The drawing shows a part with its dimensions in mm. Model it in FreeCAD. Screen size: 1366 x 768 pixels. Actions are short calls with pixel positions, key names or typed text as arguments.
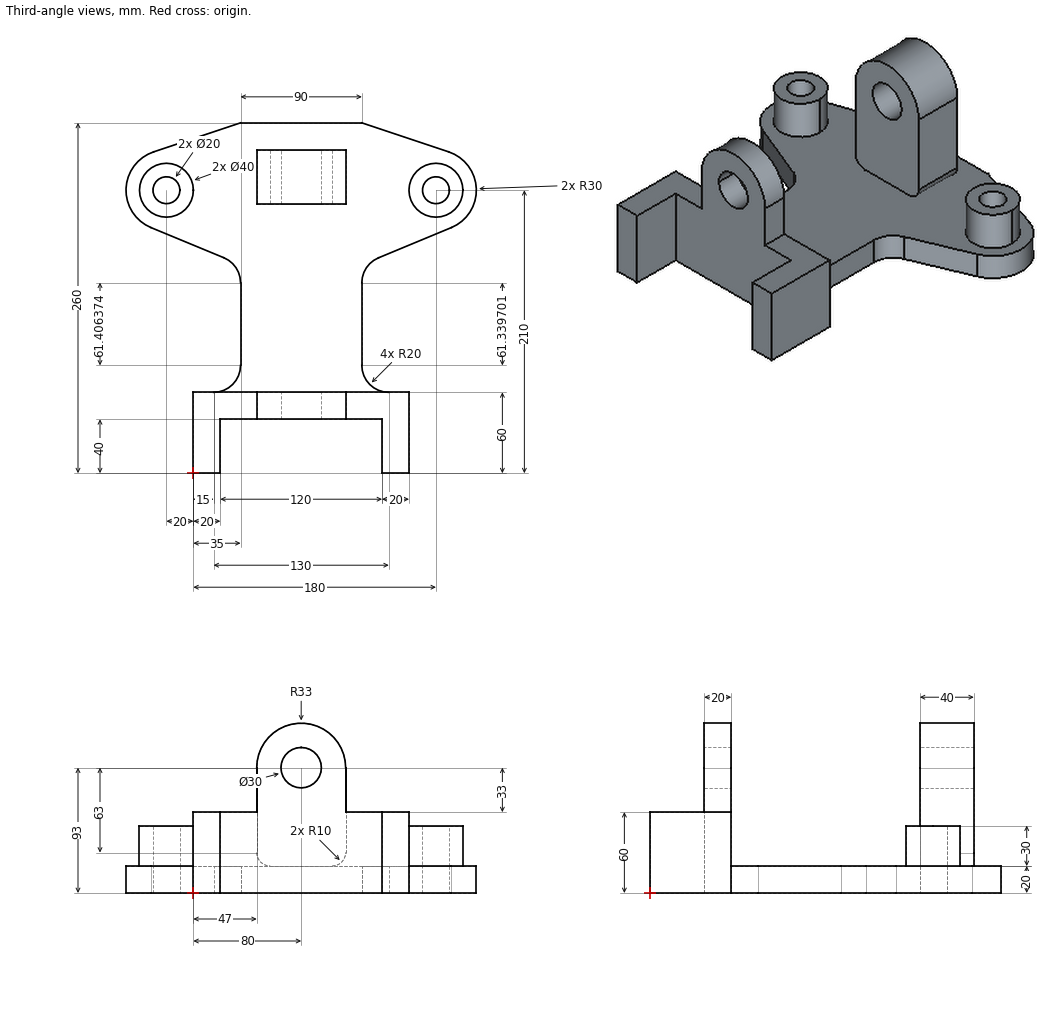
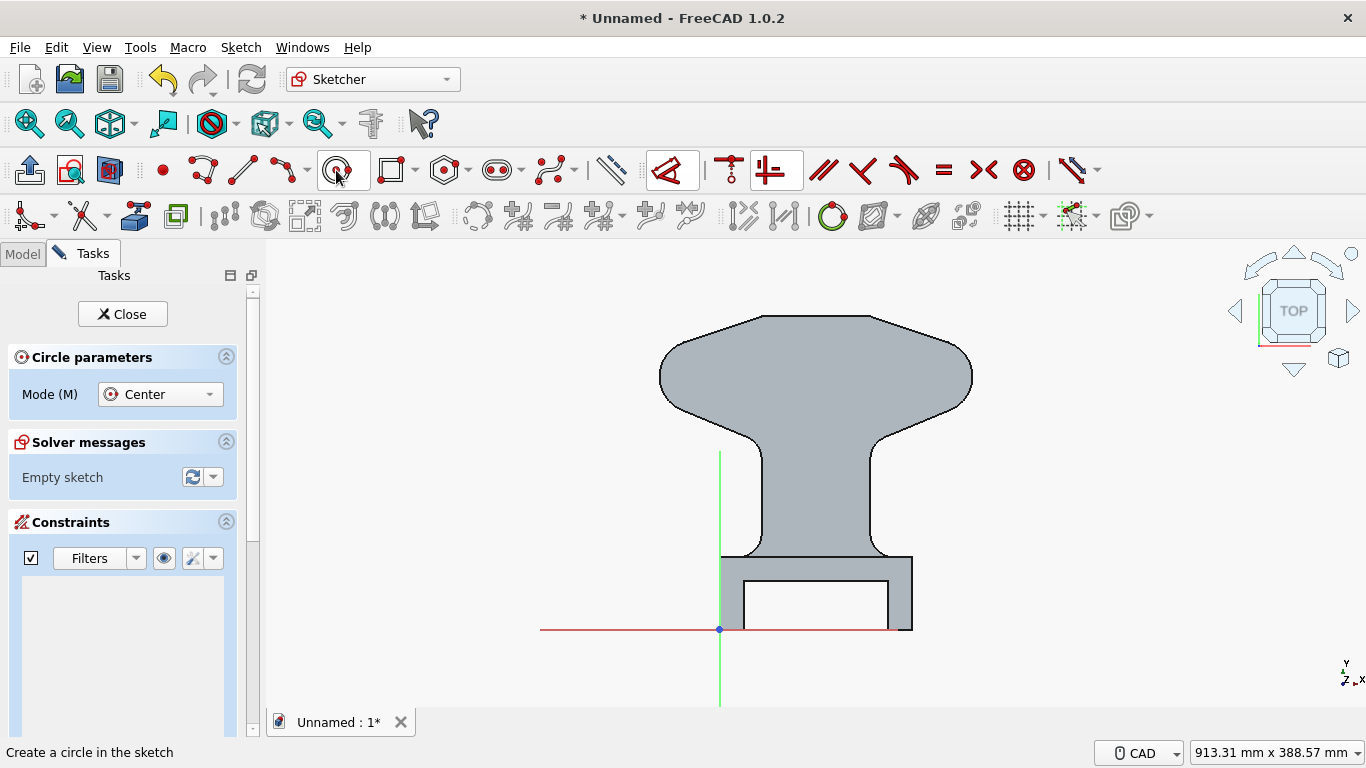
click(696, 377)
click(679, 360)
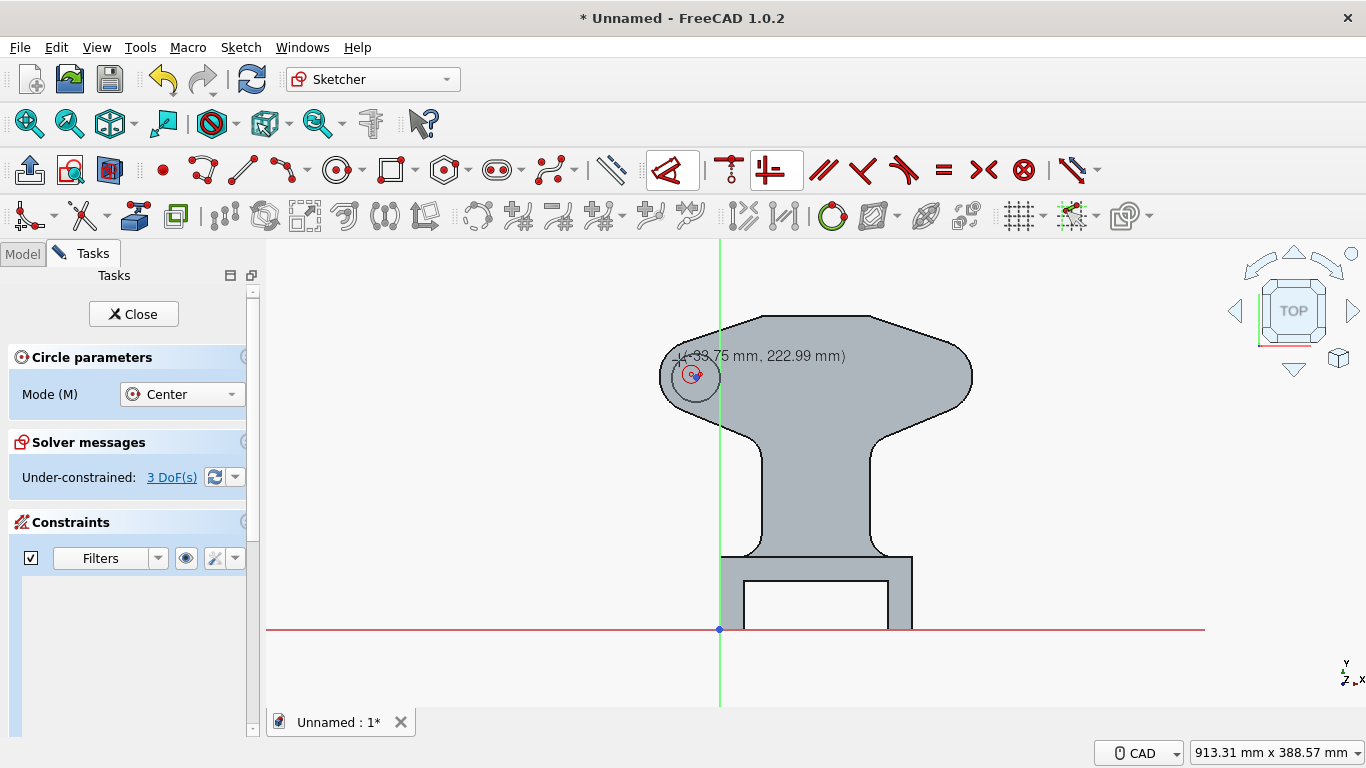
click(936, 377)
click(953, 360)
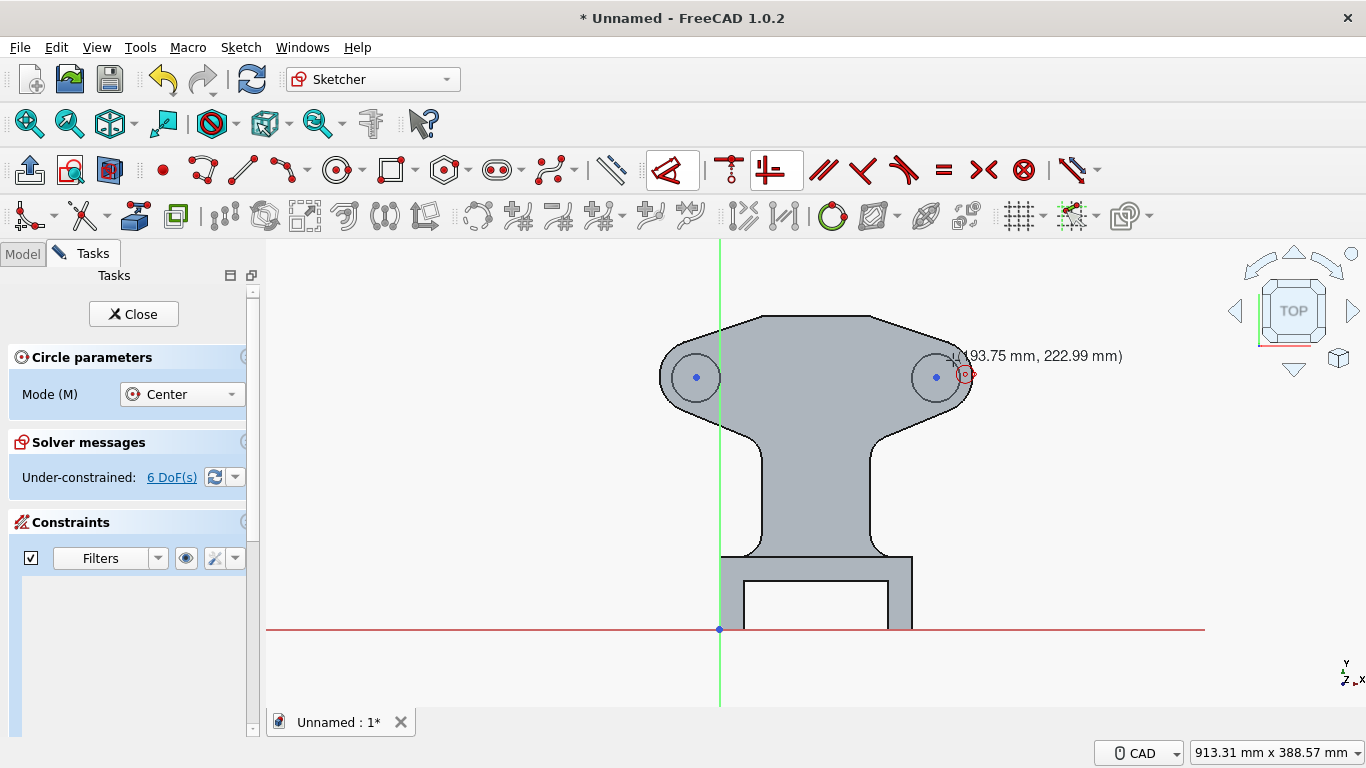
scroll(696, 377, up, 4)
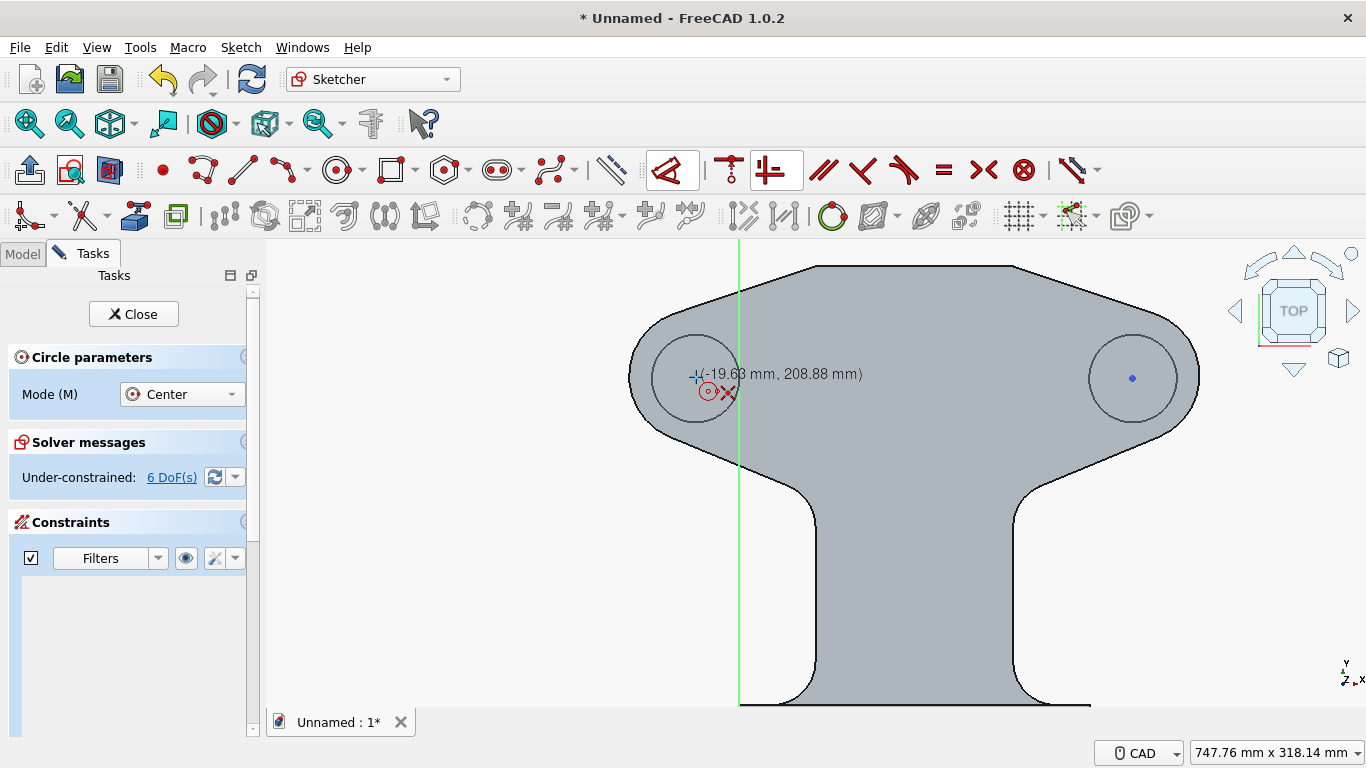
click(696, 379)
click(713, 357)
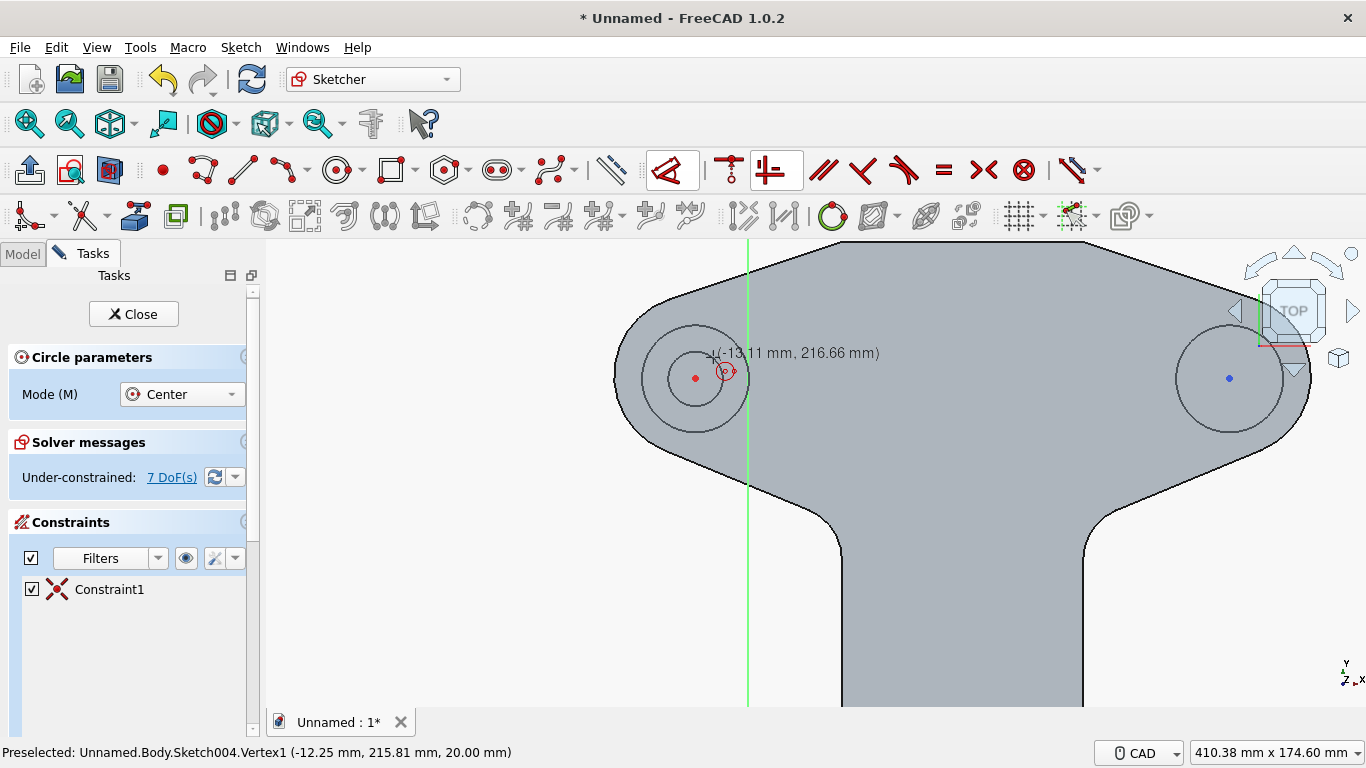
scroll(572, 344, down, 4)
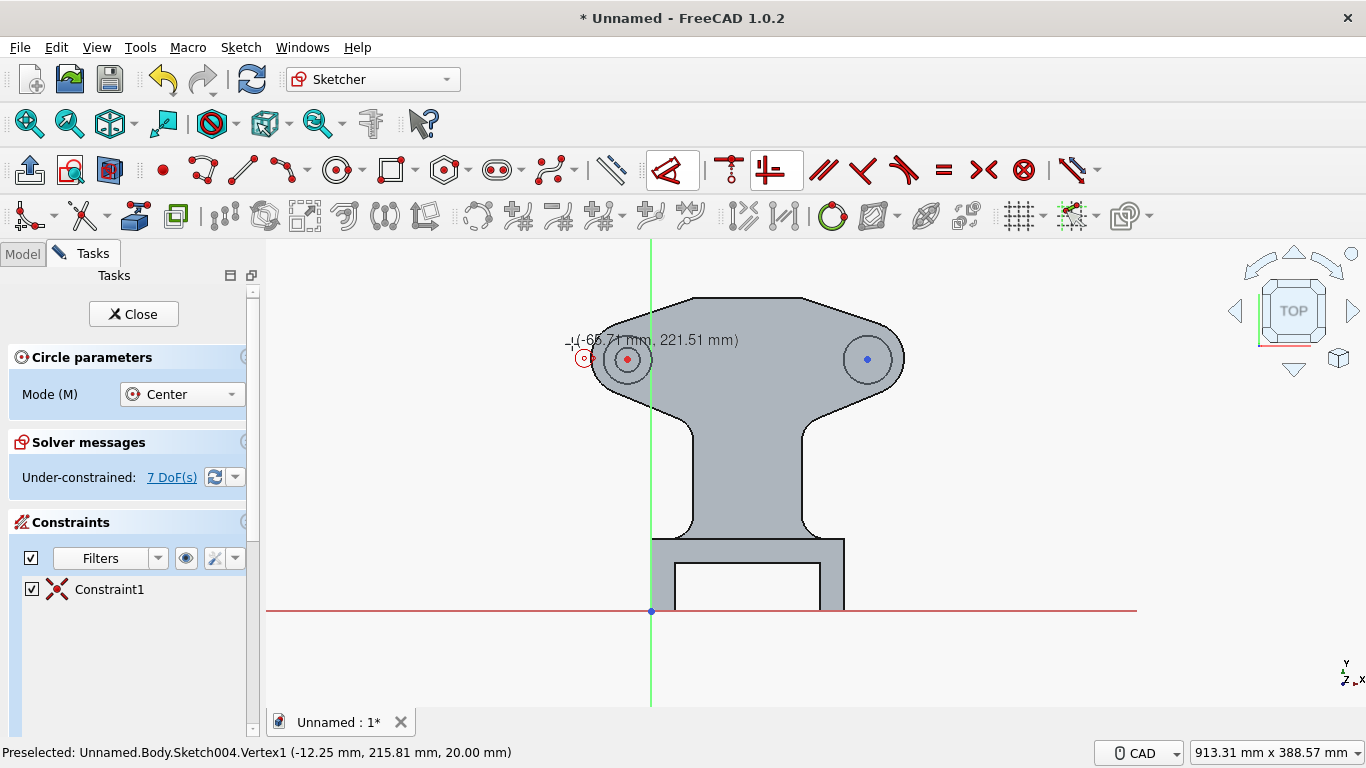
scroll(868, 358, up, 4)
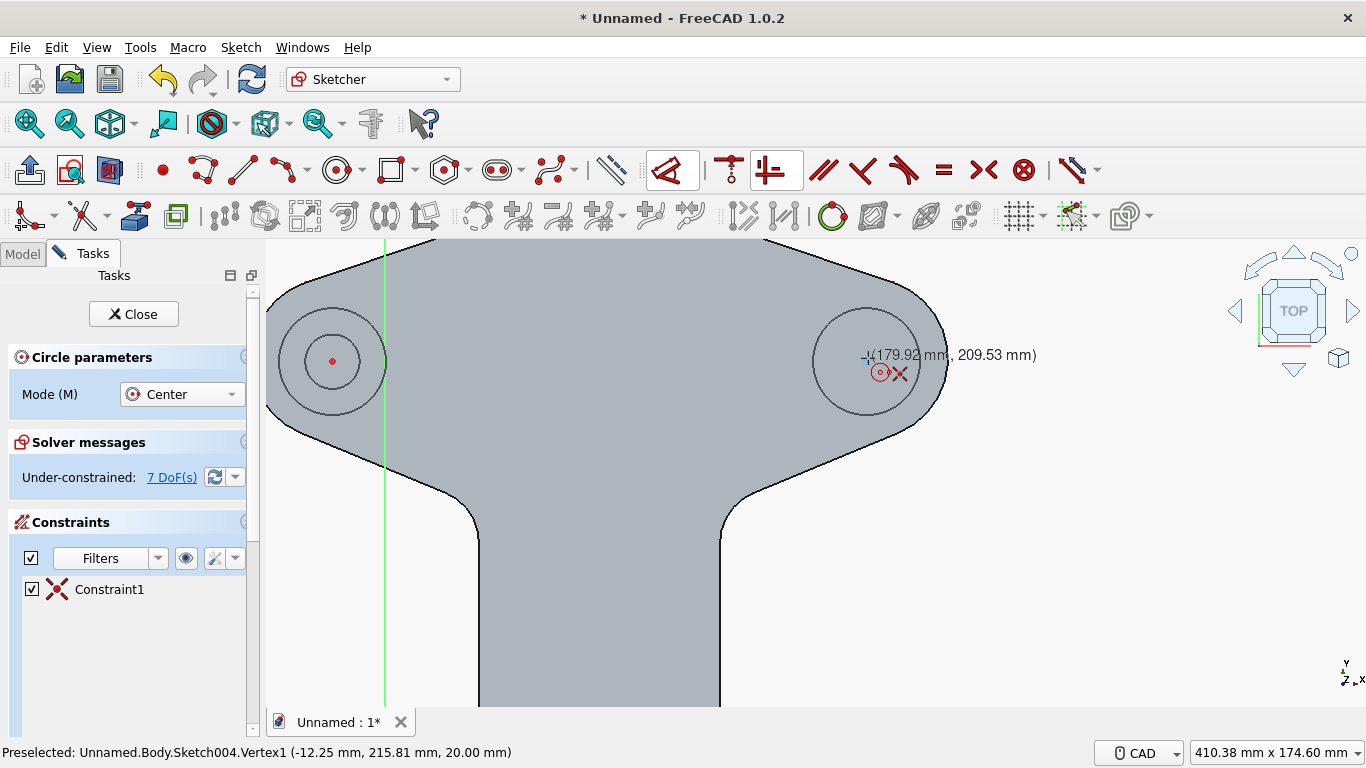
click(867, 362)
click(886, 340)
key(Escape)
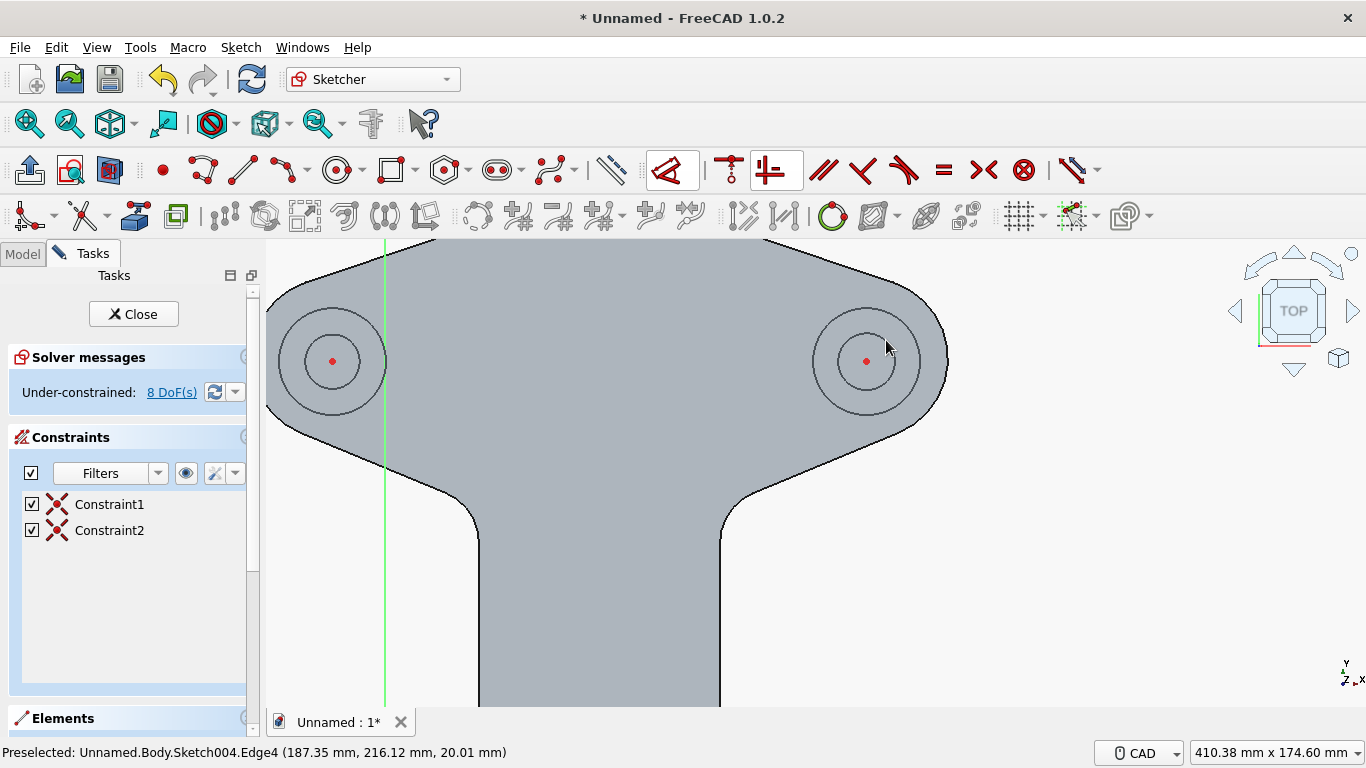
click(370, 324)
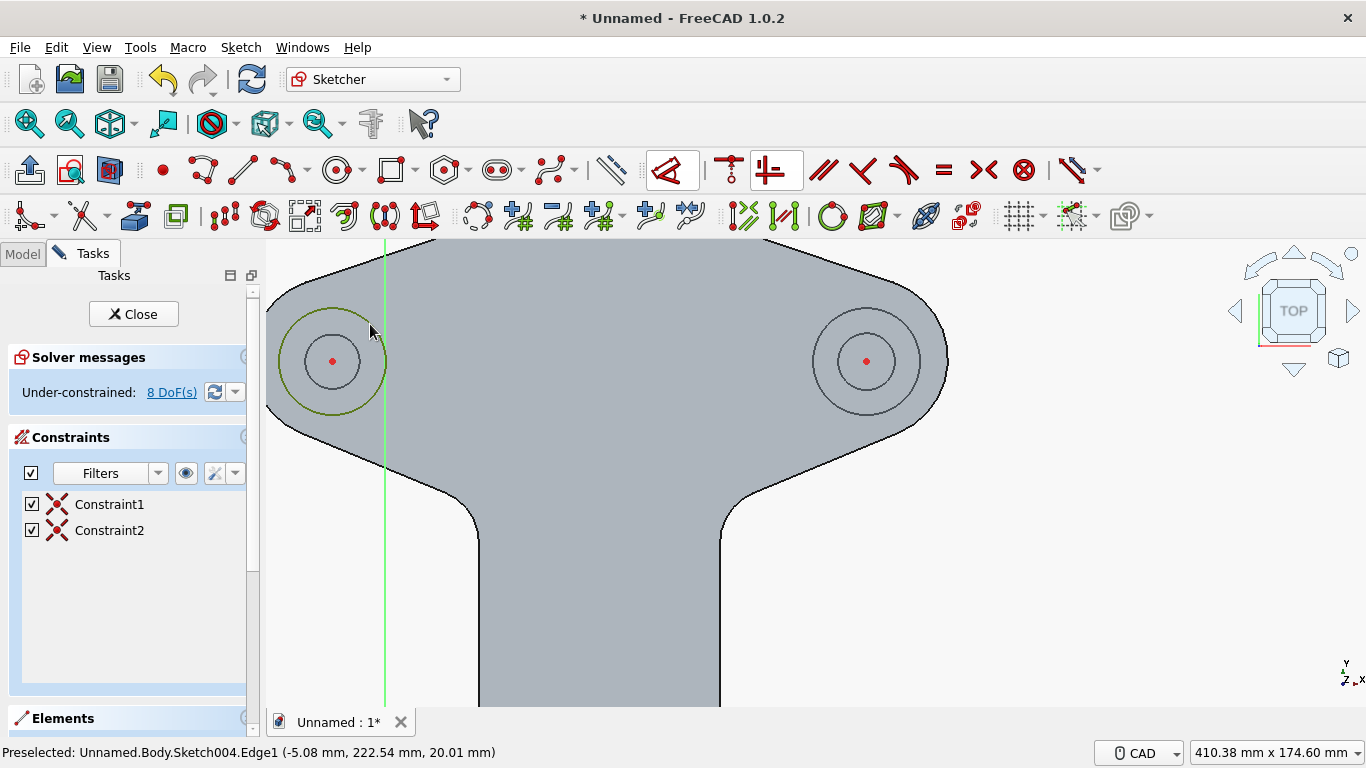
click(904, 324)